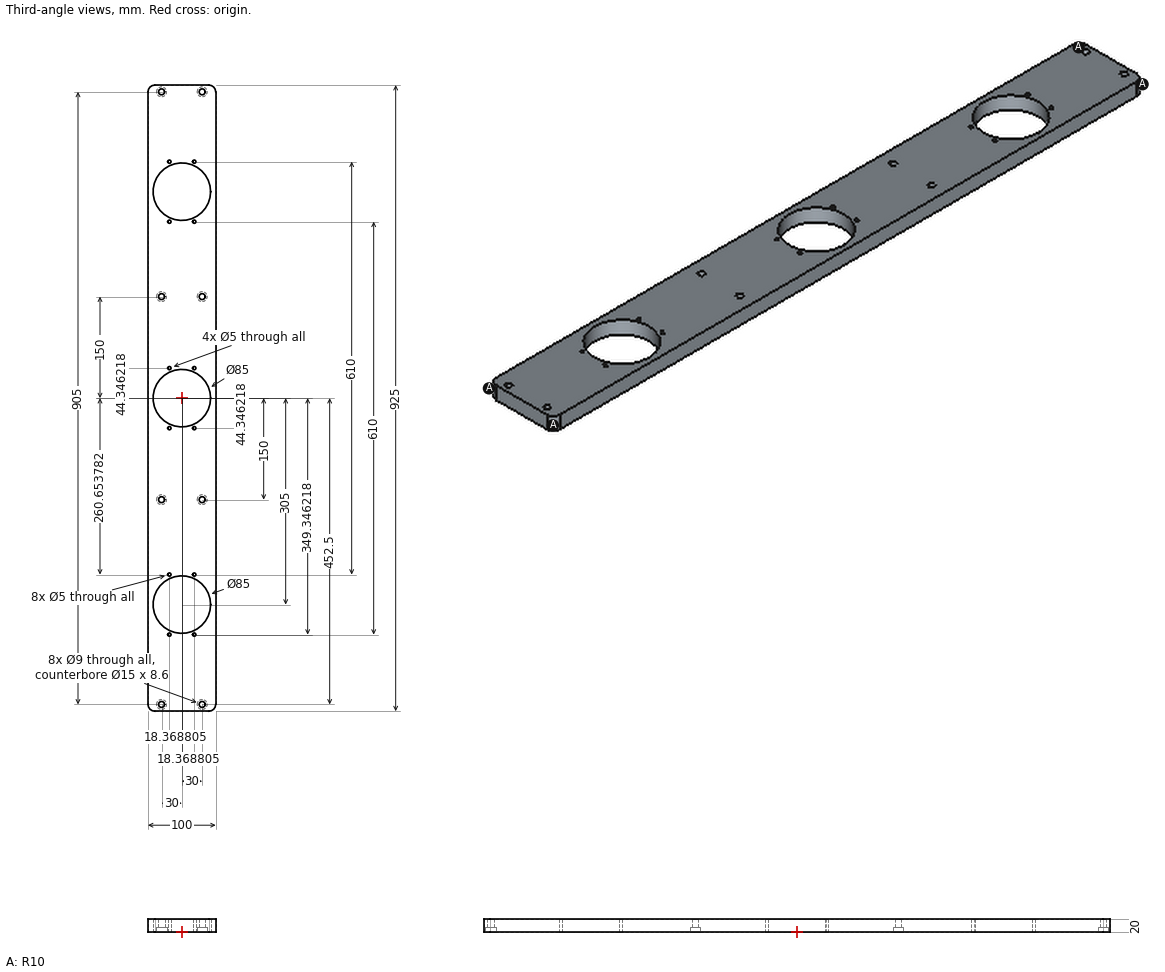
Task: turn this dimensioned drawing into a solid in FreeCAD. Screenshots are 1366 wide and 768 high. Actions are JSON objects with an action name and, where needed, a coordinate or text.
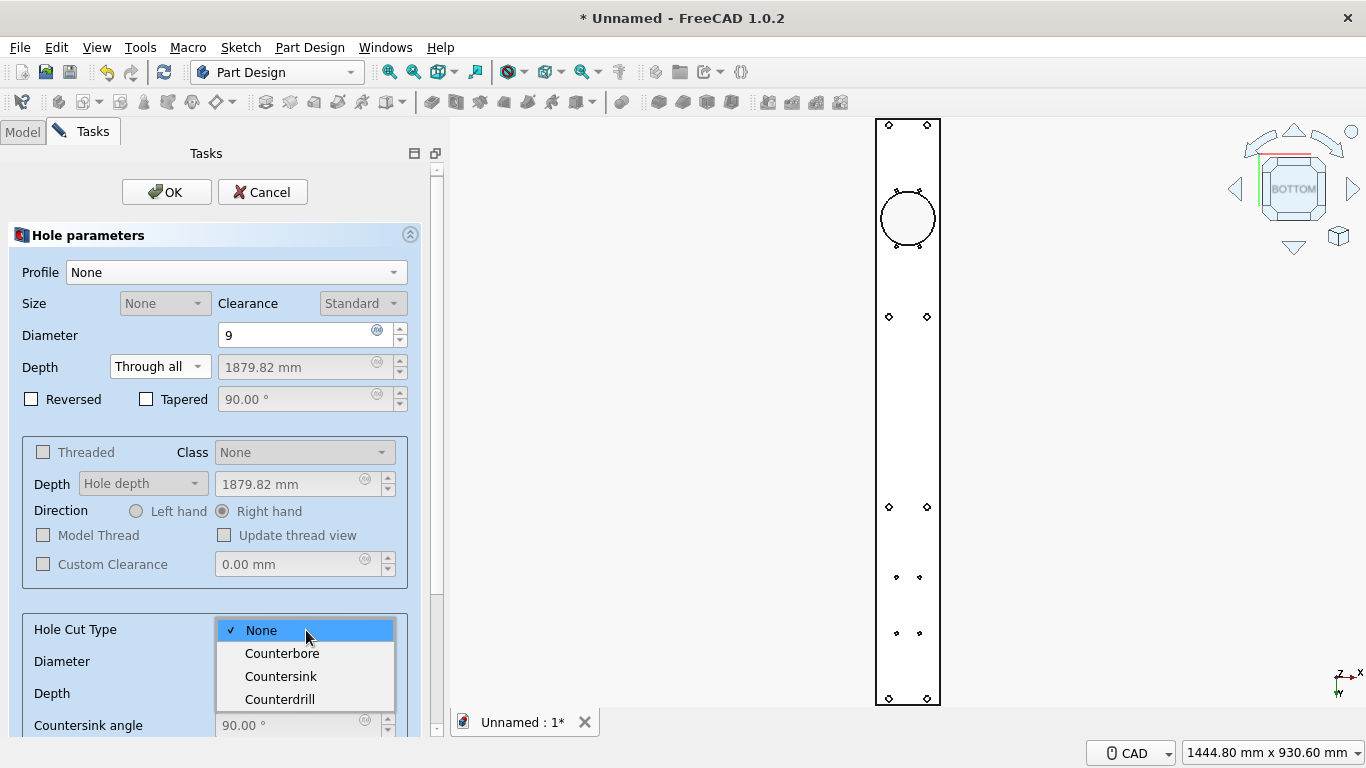
{"action": "left_click", "coordinate": [304, 654]}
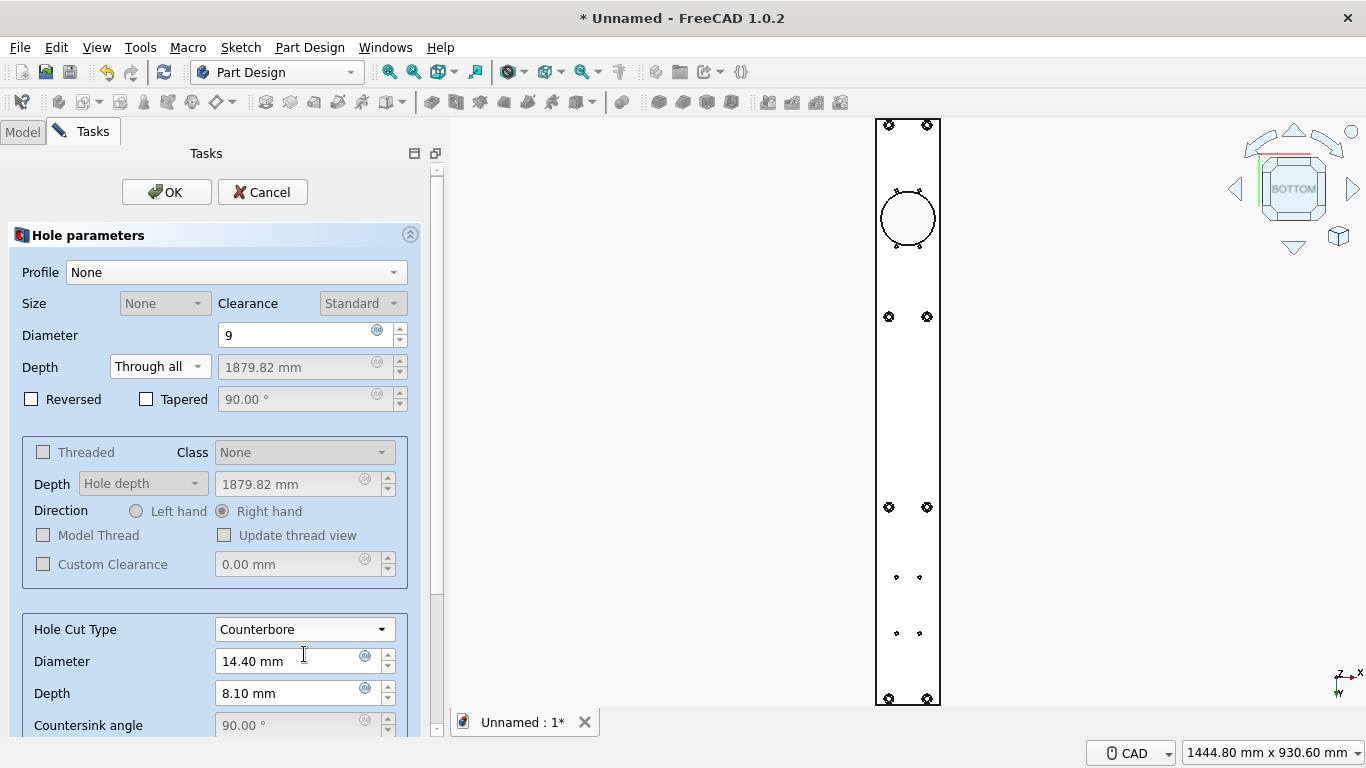
{"action": "triple_click", "coordinate": [298, 661]}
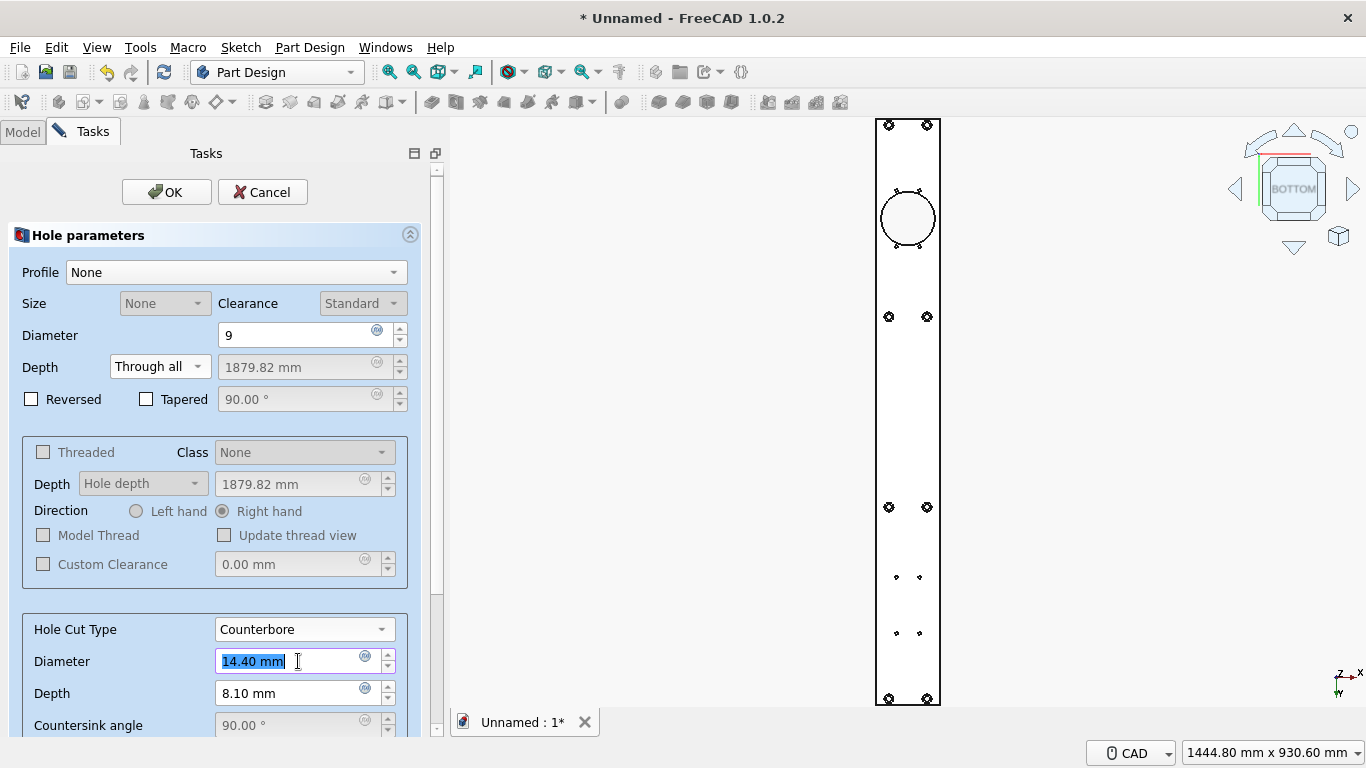
{"action": "type", "text": "15"}
{"action": "key", "text": "Tab"}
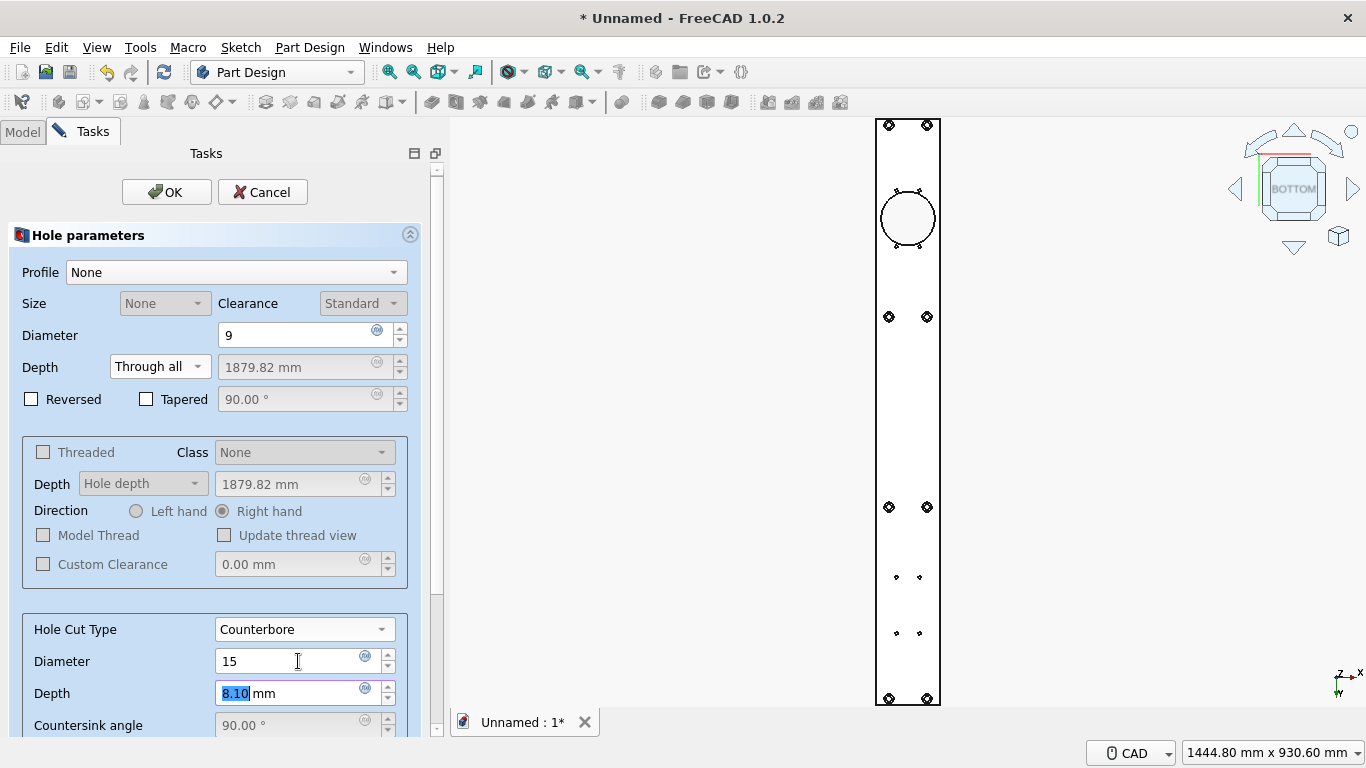
{"action": "type", "text": "8.6"}
{"action": "key", "text": "Tab"}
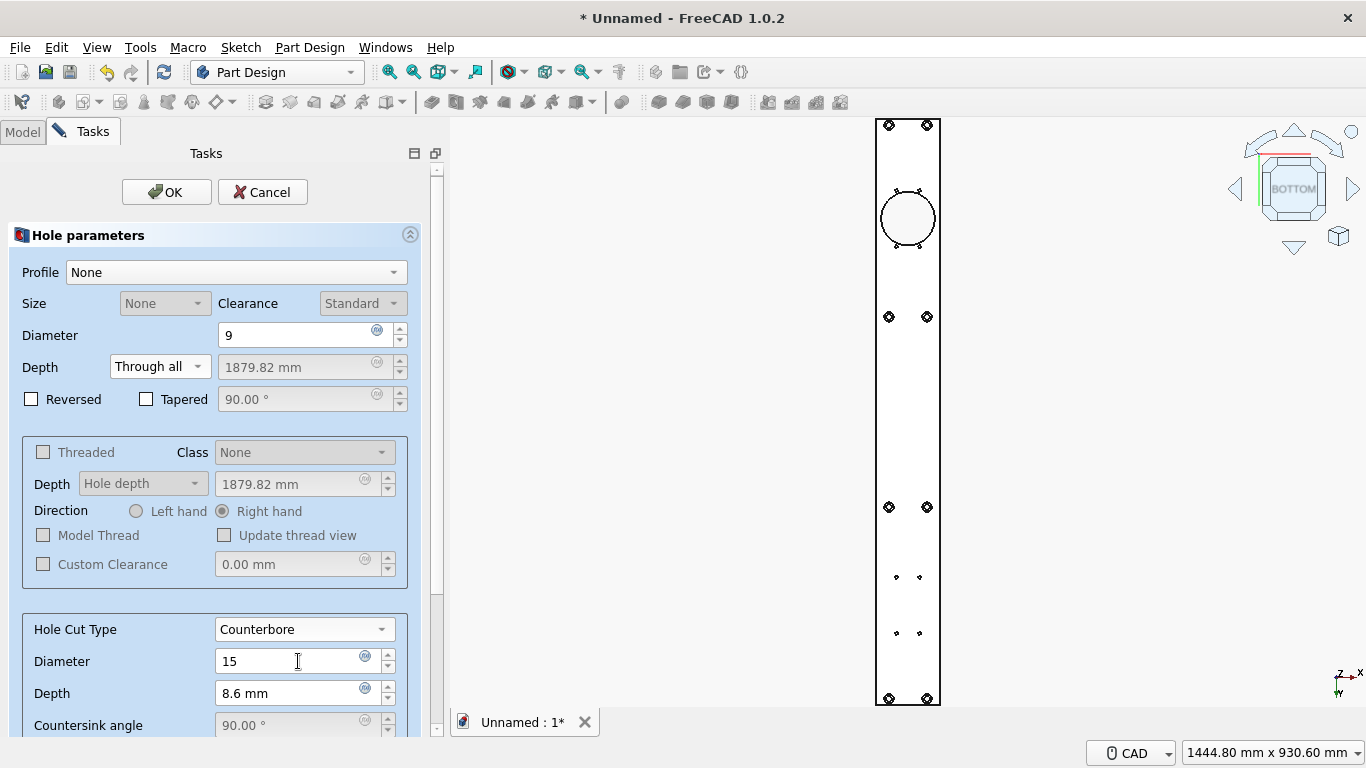
{"action": "left_click", "coordinate": [167, 192]}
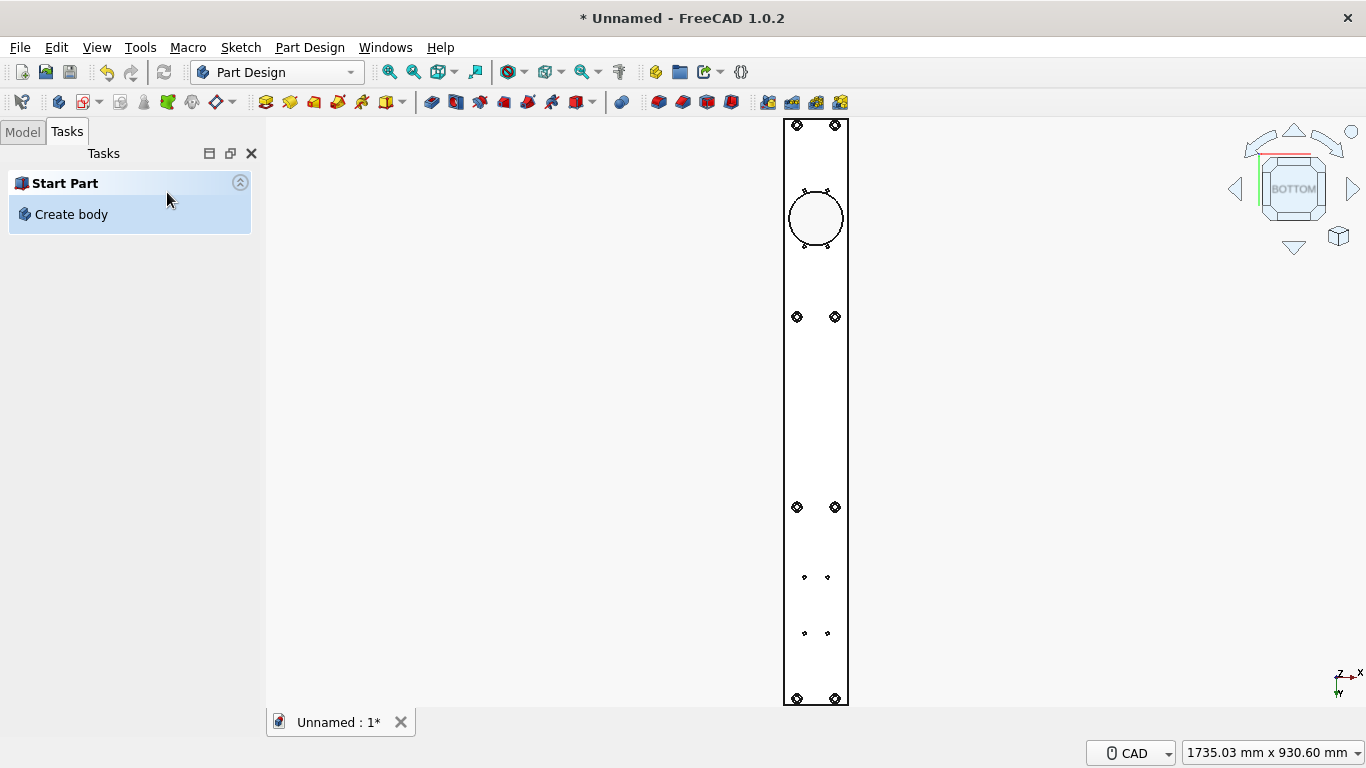
{"action": "left_click", "coordinate": [23, 131]}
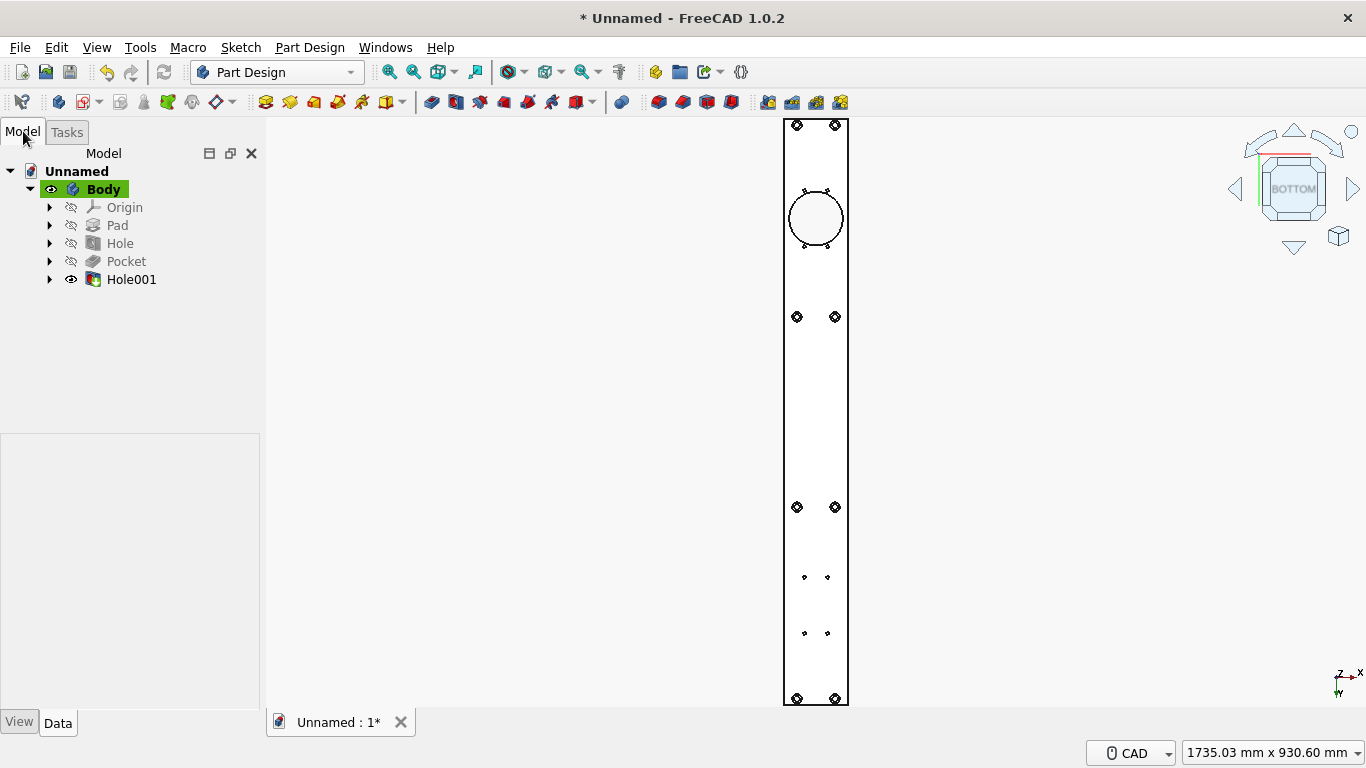
{"action": "left_click", "coordinate": [116, 261]}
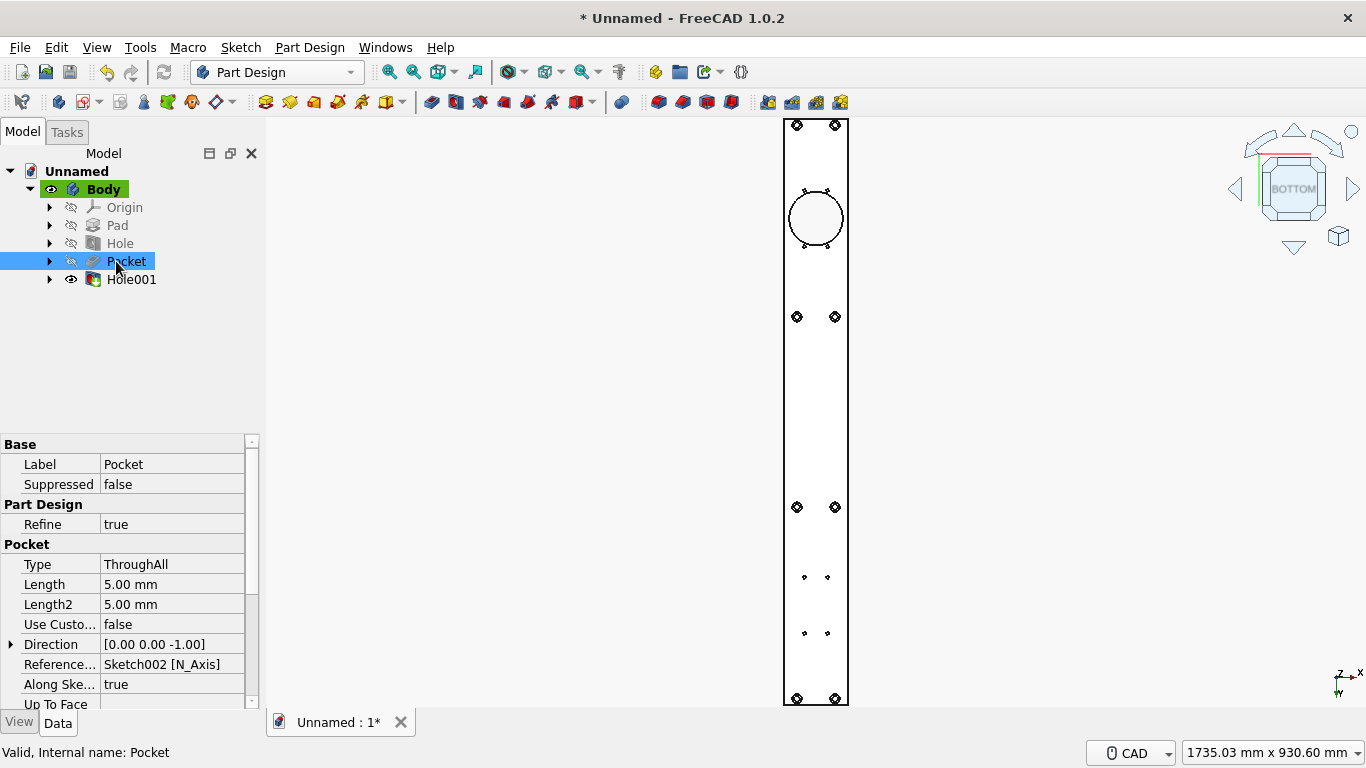
{"action": "left_click", "coordinate": [768, 102]}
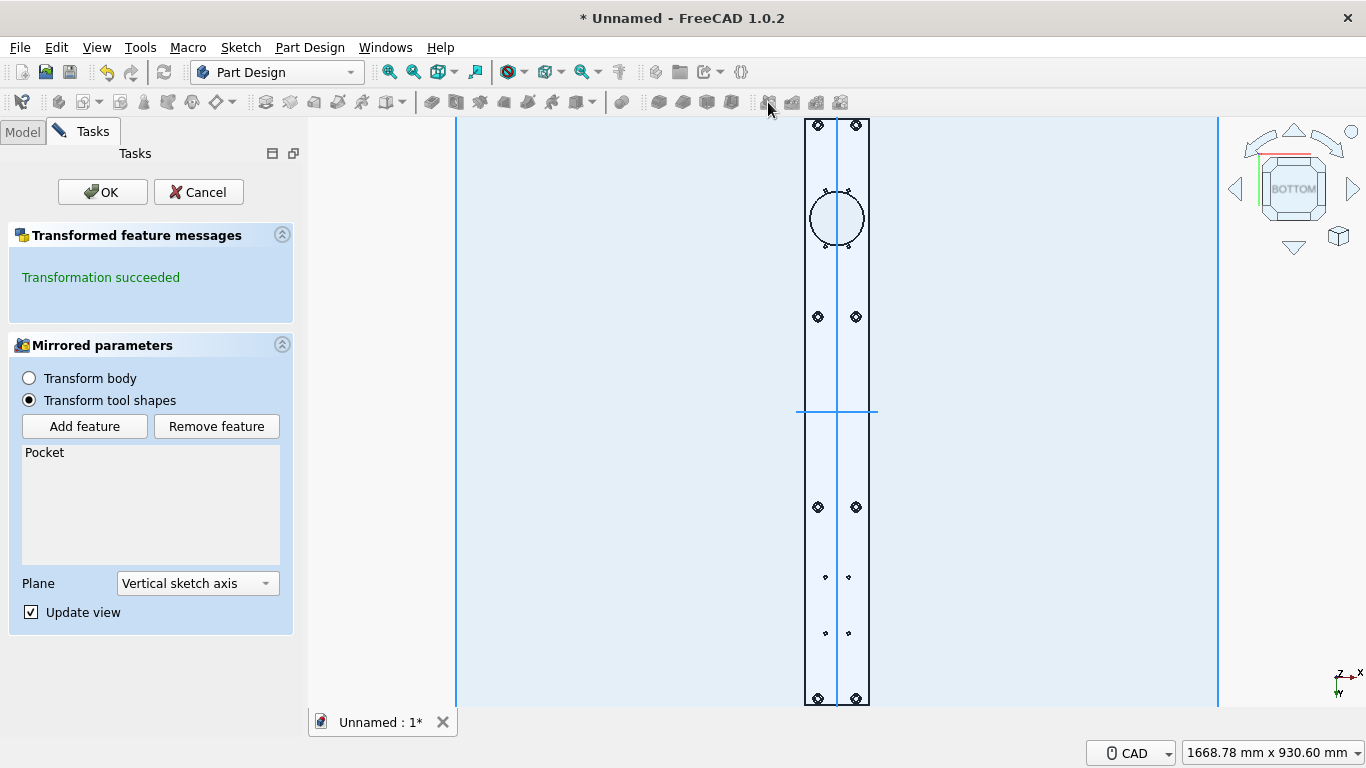
{"action": "left_click", "coordinate": [198, 584]}